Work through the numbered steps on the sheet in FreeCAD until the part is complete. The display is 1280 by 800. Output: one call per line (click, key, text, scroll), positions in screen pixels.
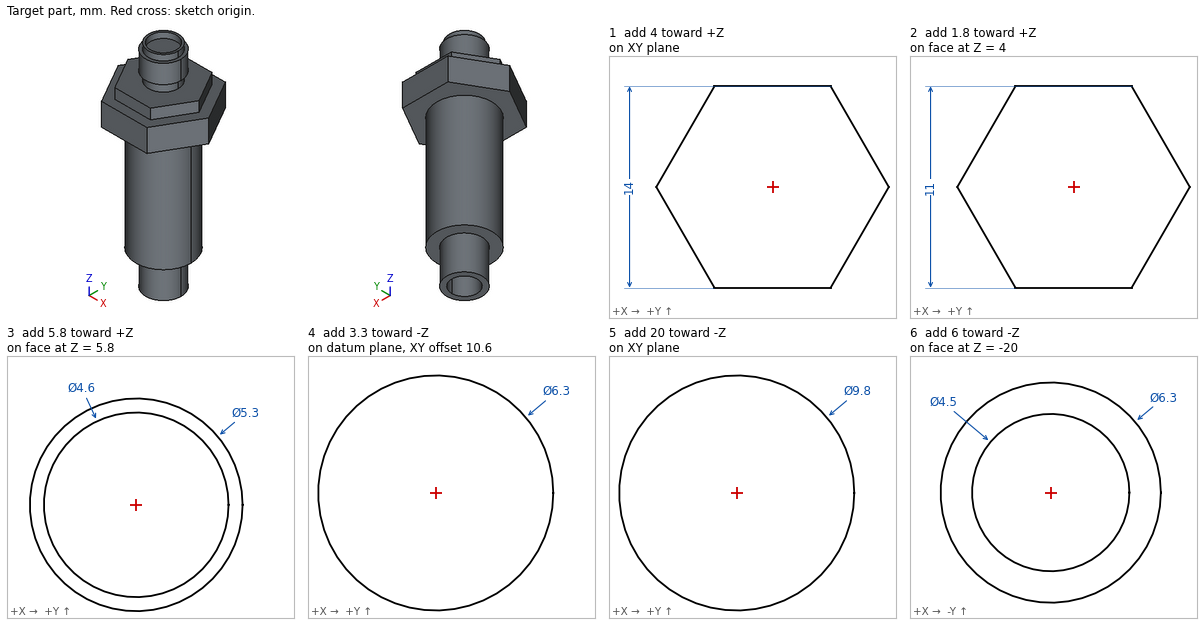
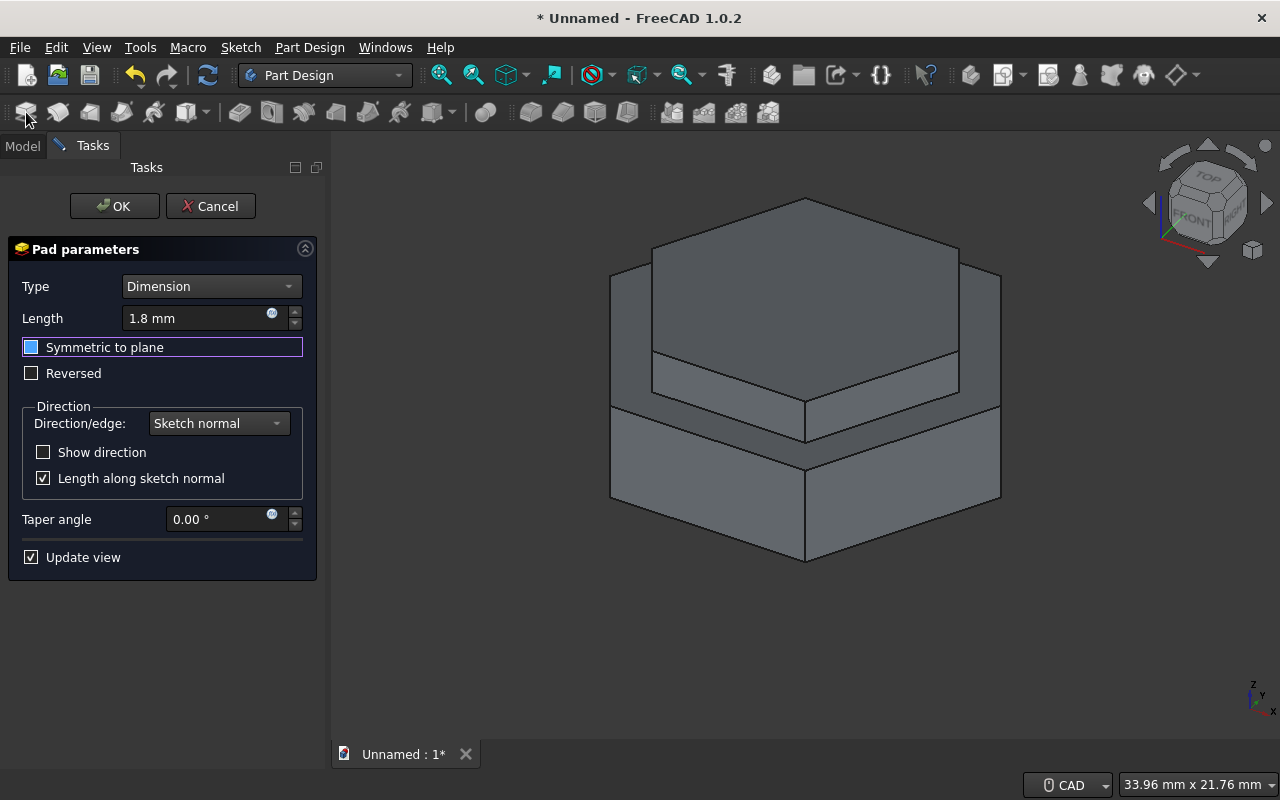
click(115, 206)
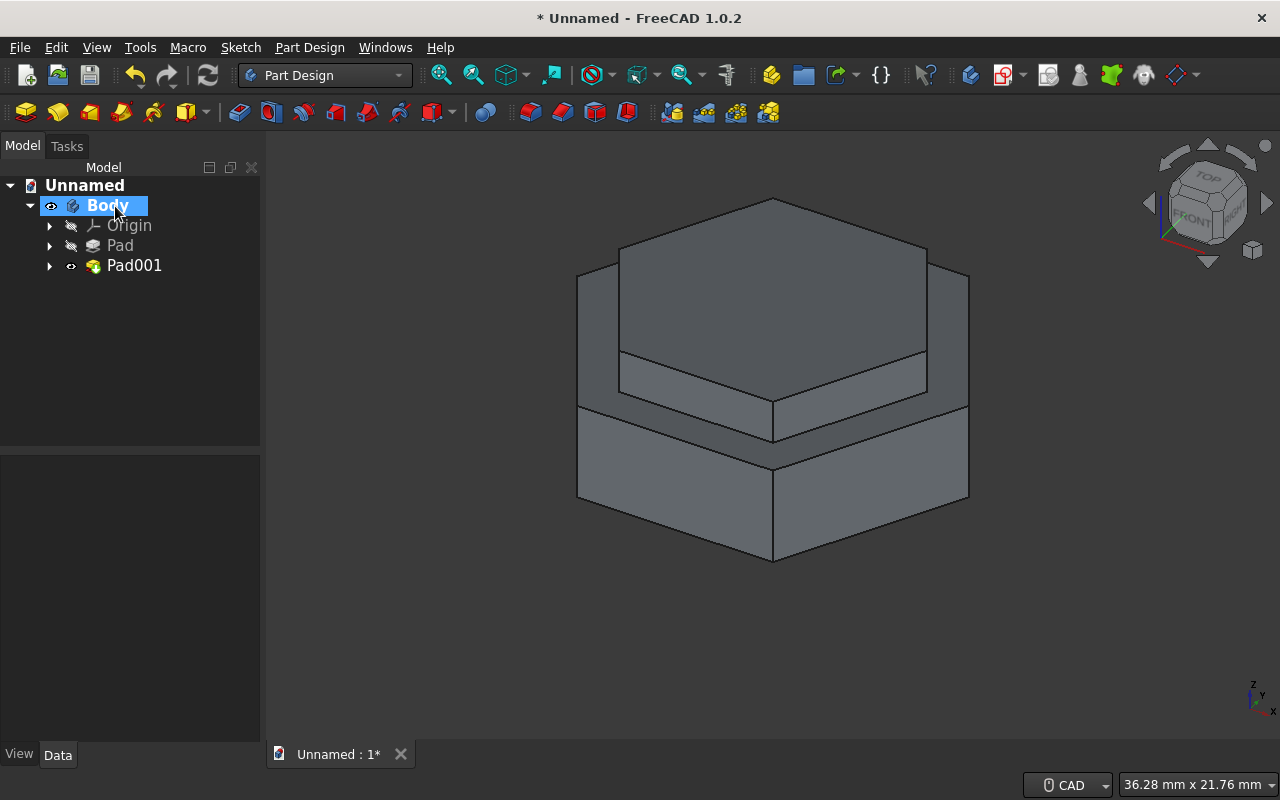
click(773, 299)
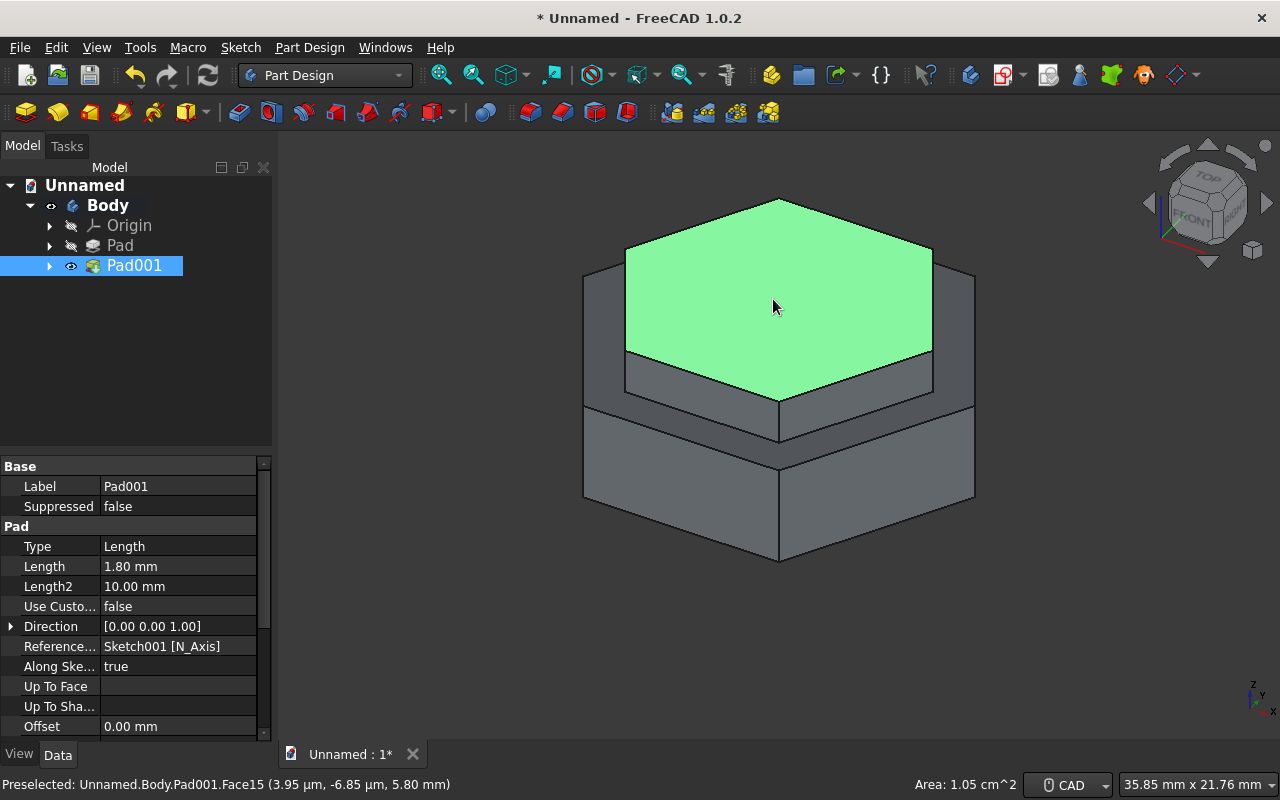
click(1004, 76)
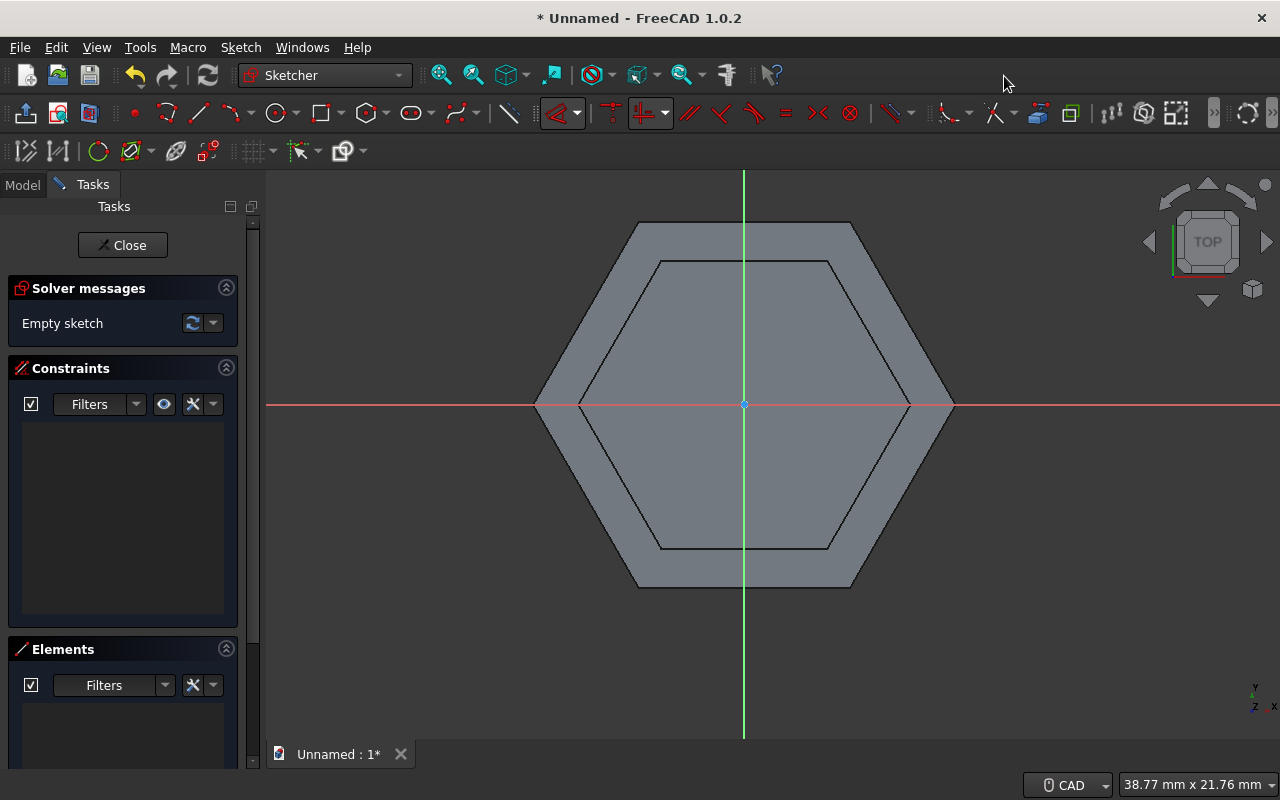
scroll(768, 376, up, 5)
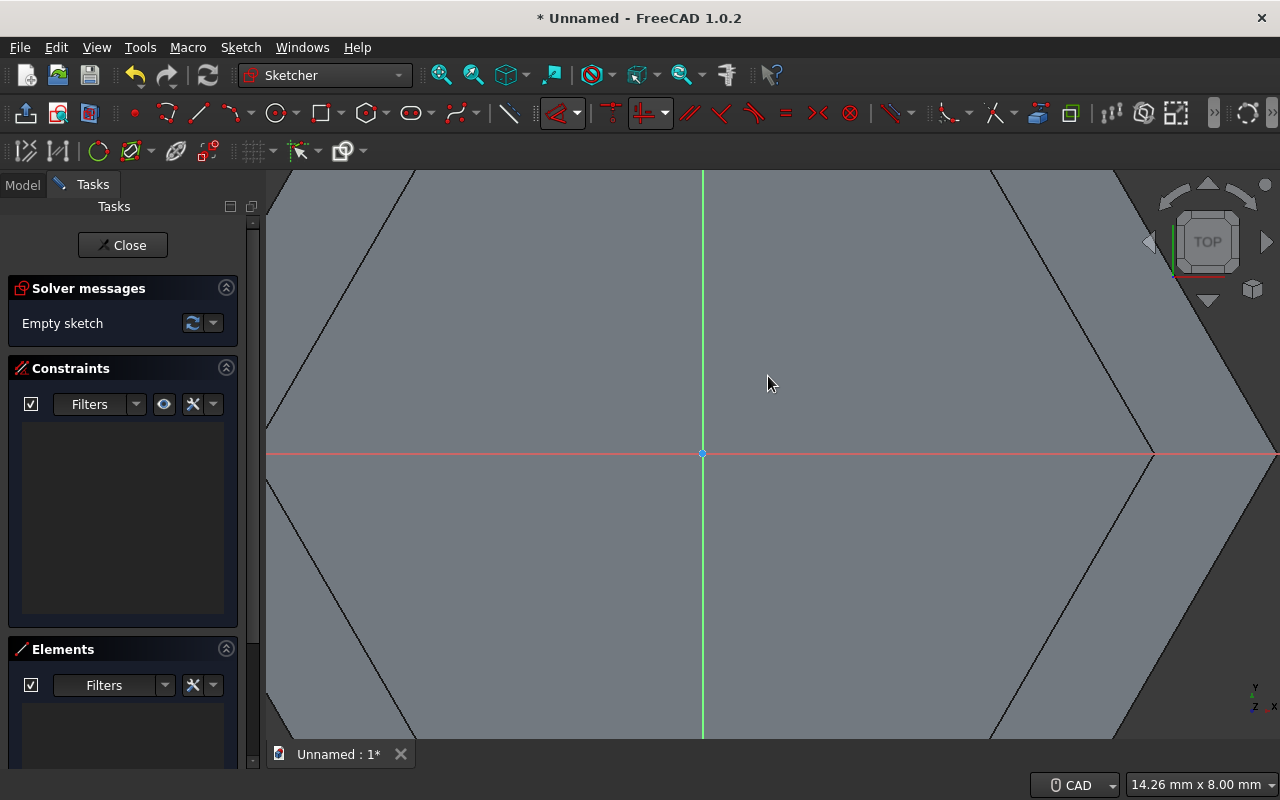
click(276, 114)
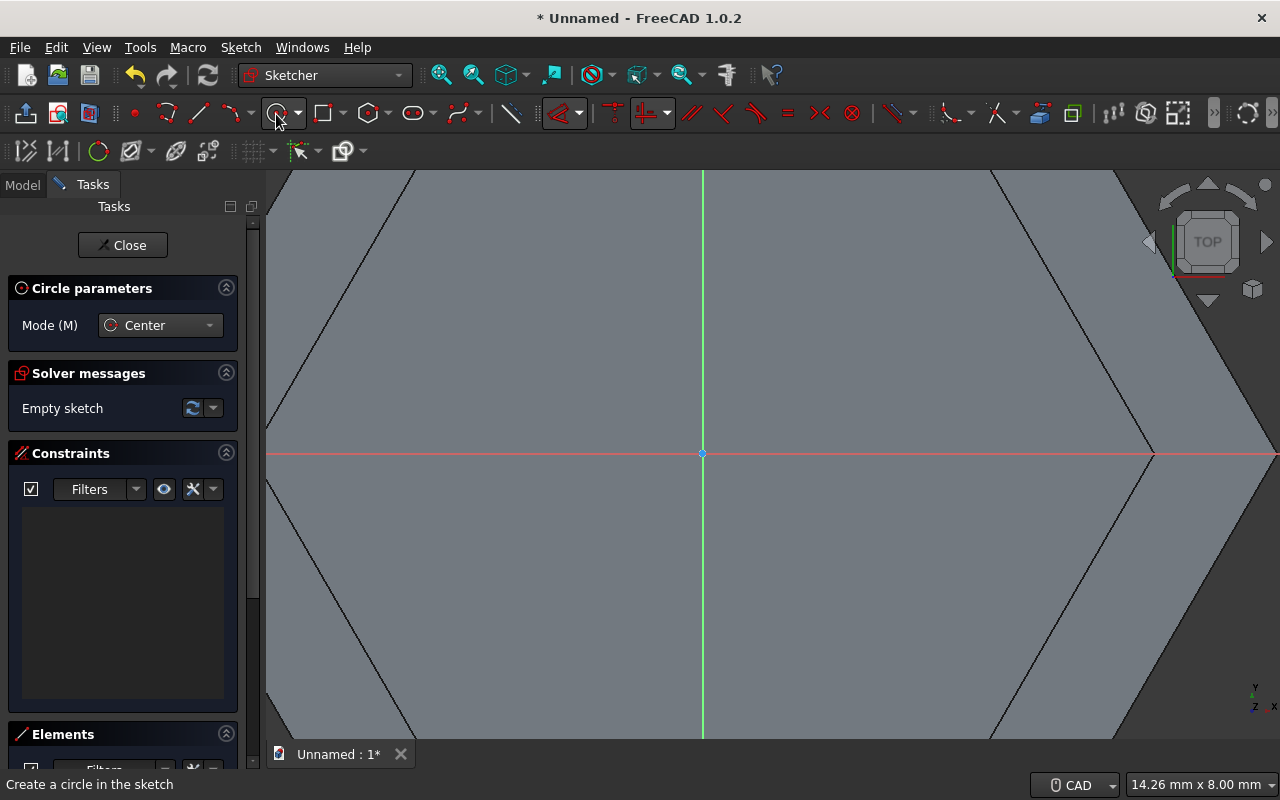
click(703, 454)
click(836, 321)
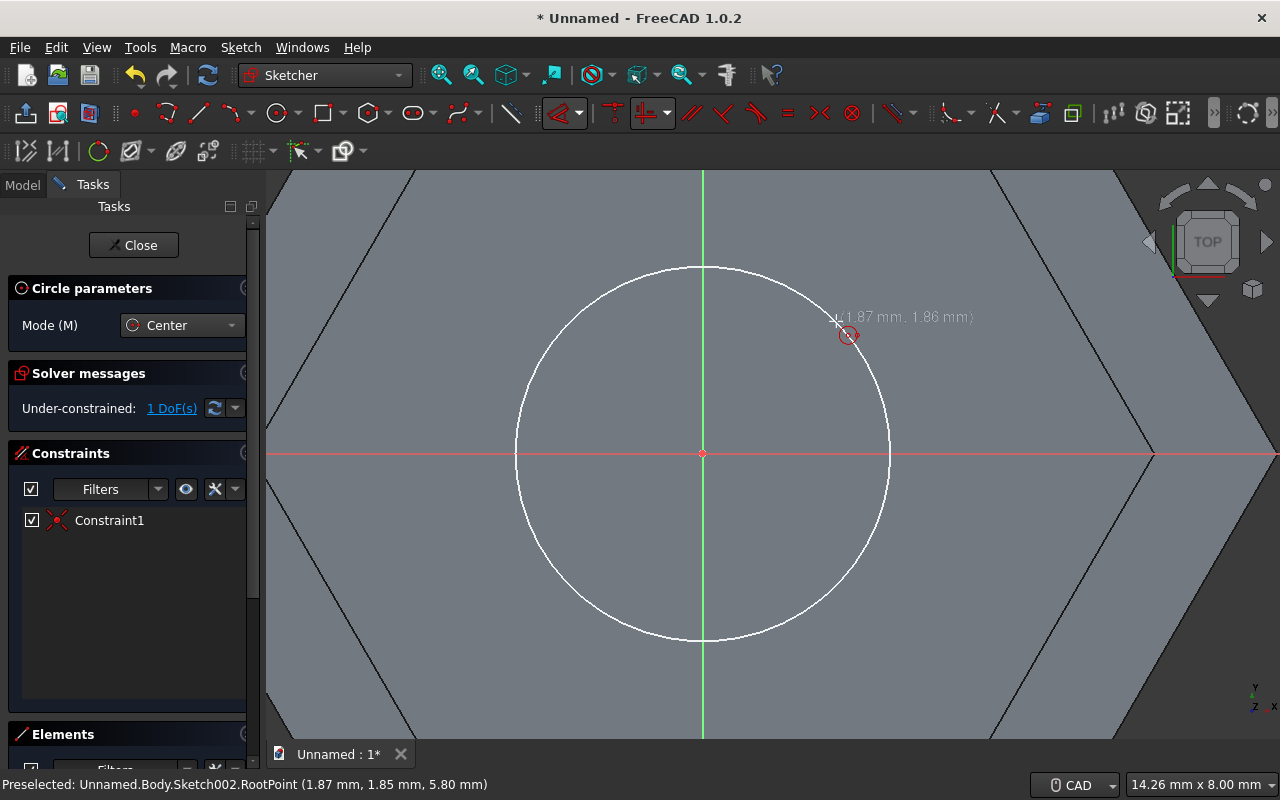
click(703, 454)
click(819, 338)
key(Escape)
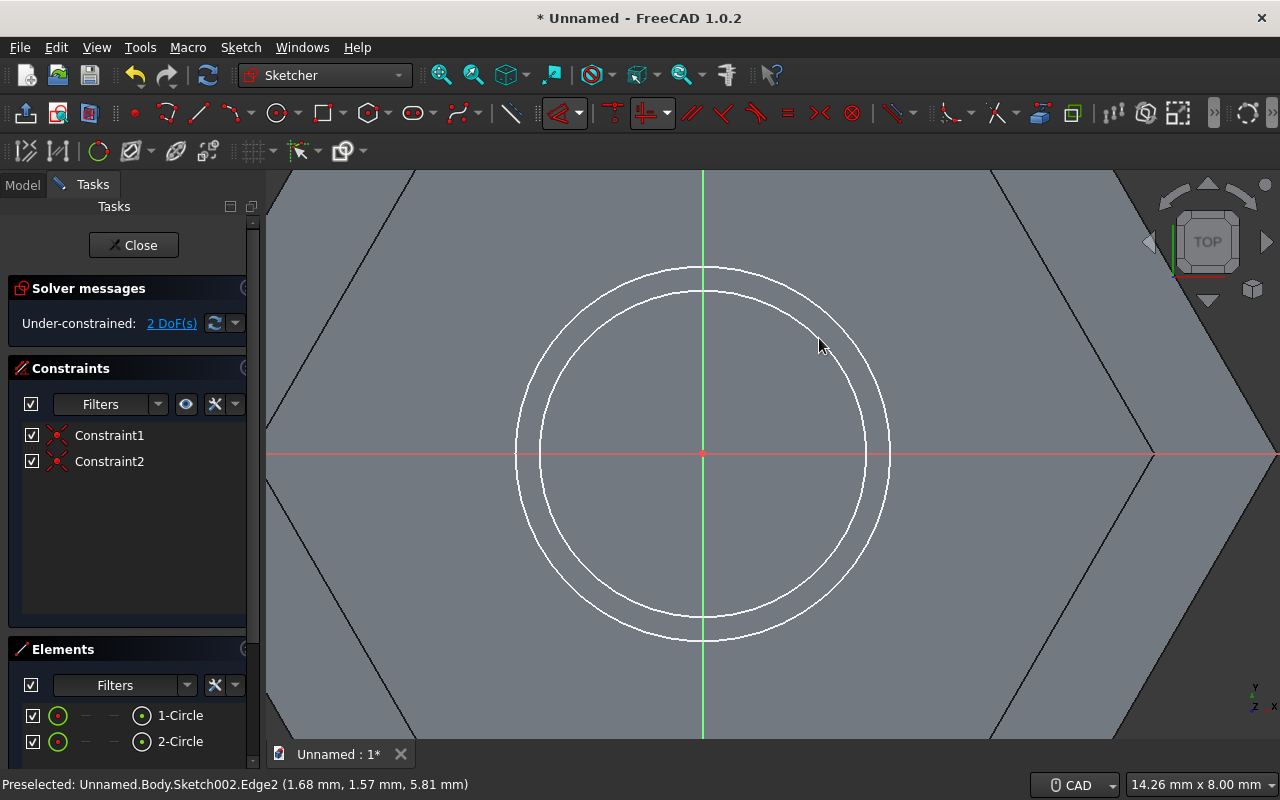
click(835, 321)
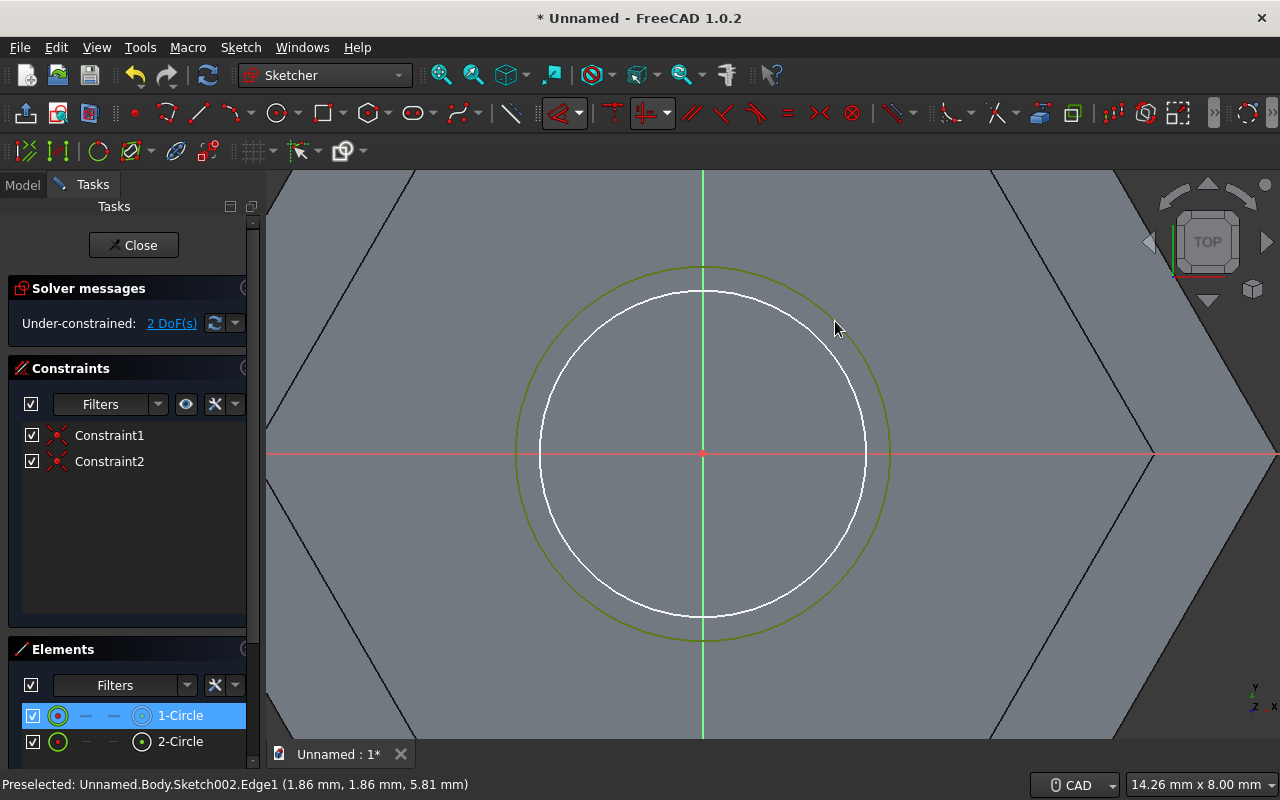
click(582, 114)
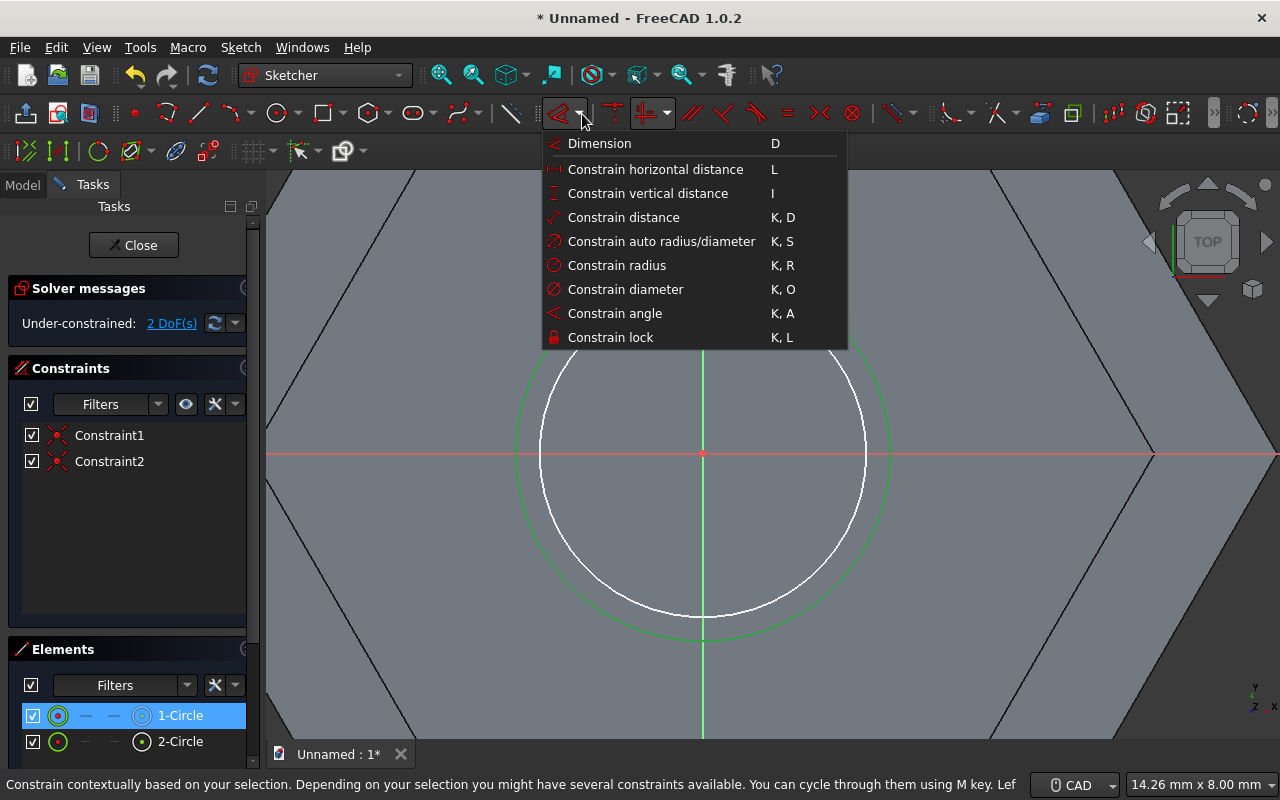
click(695, 289)